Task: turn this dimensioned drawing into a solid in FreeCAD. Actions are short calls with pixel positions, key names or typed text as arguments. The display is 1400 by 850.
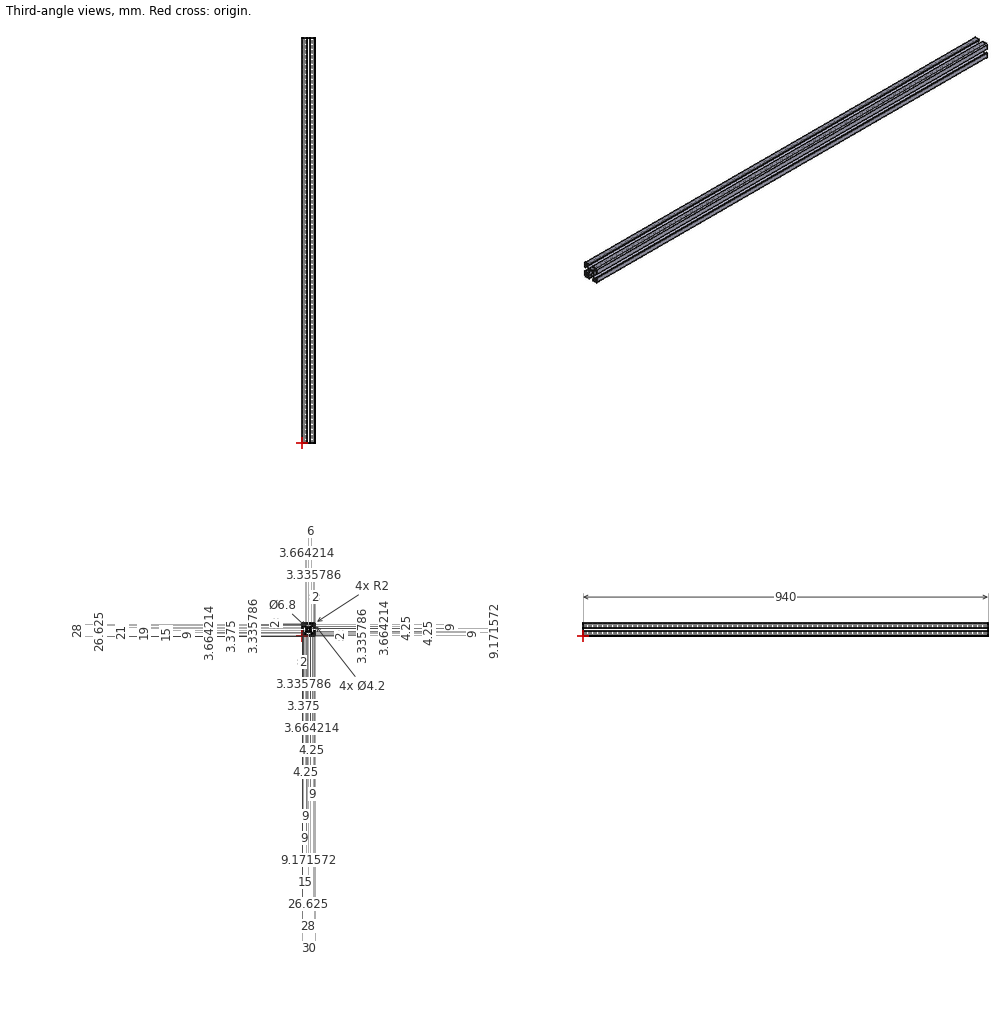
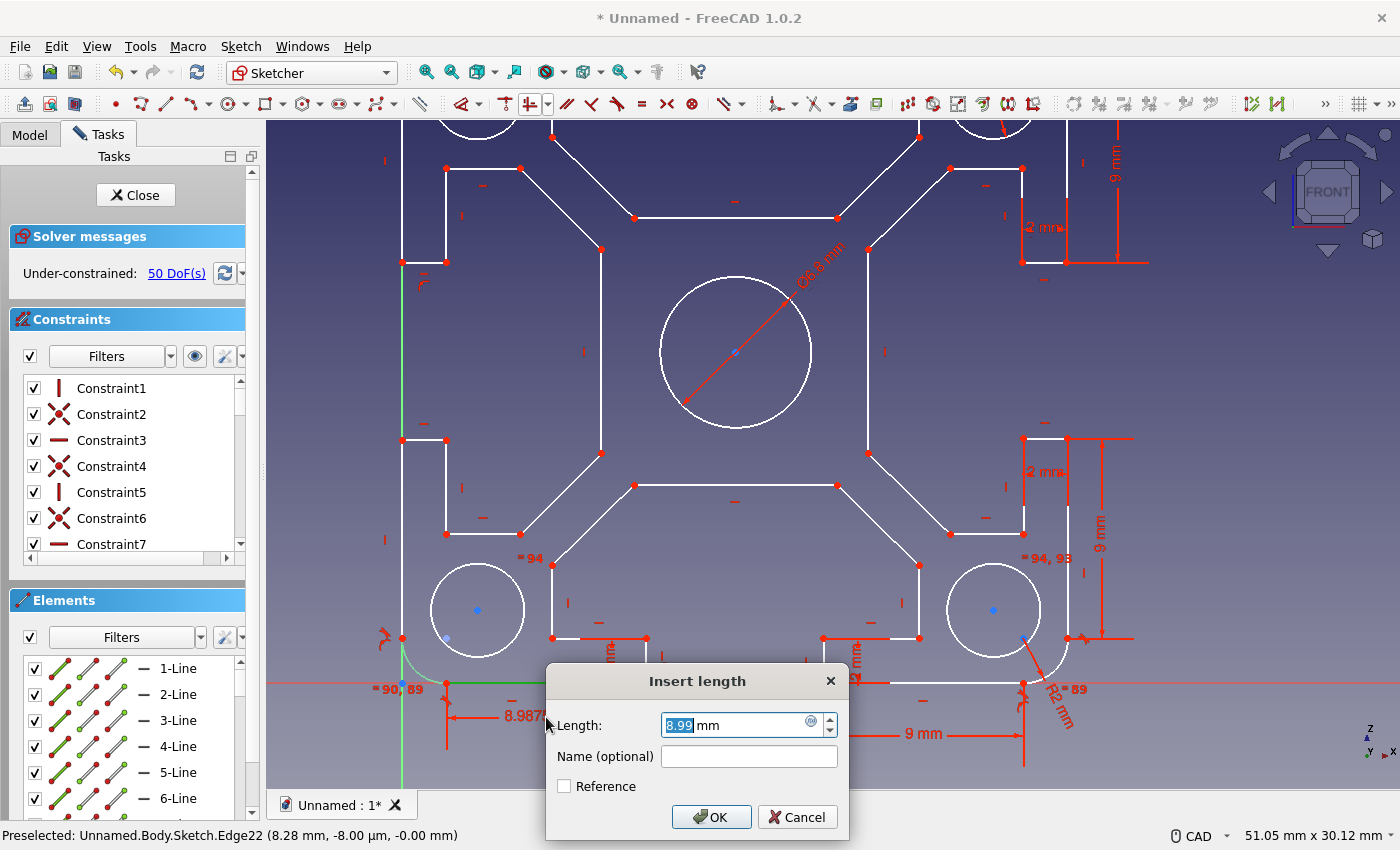
text(9)
key(Return)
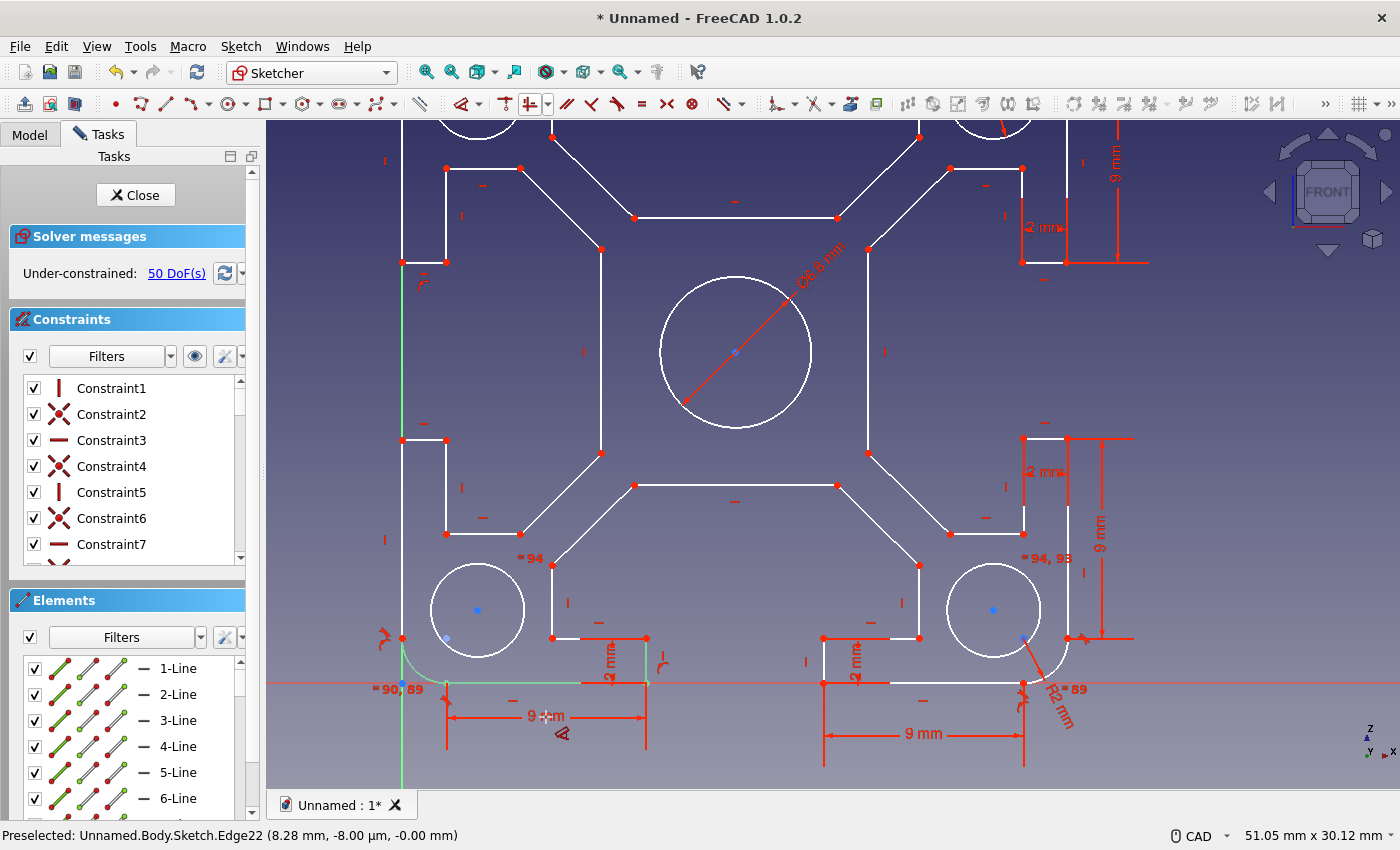
click(402, 579)
click(368, 540)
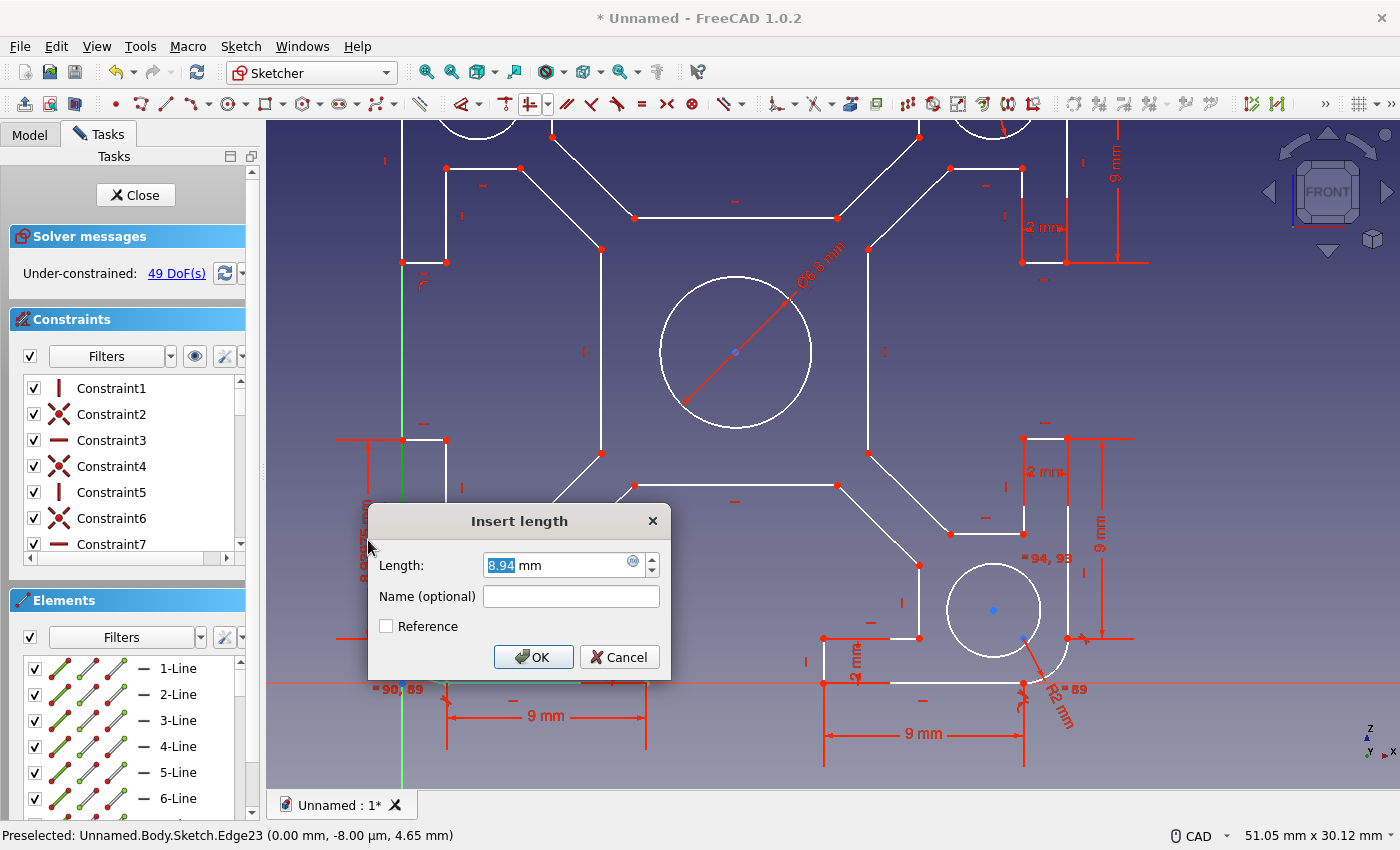
text(9)
key(Return)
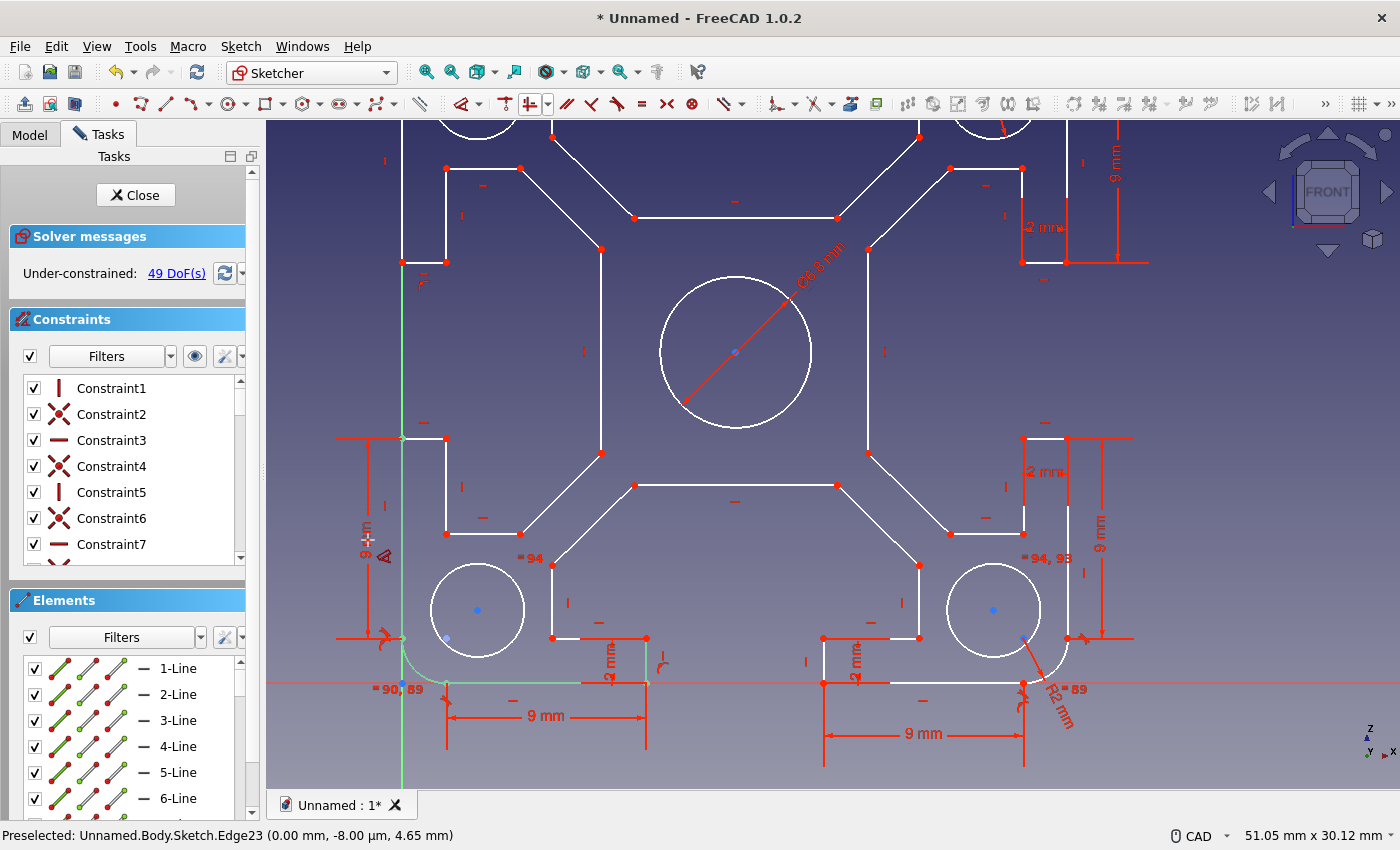
click(415, 439)
click(424, 473)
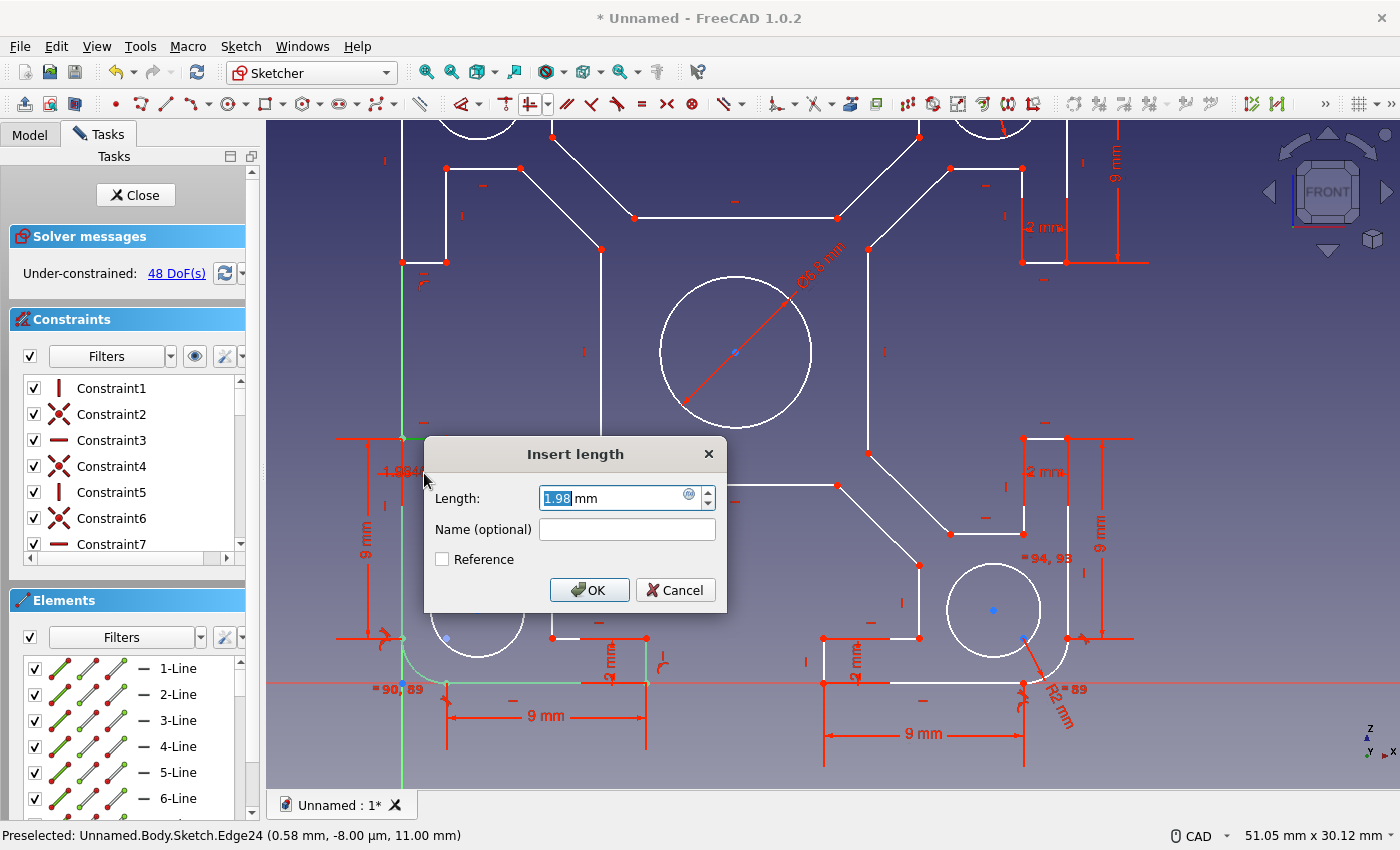
text(2)
key(Return)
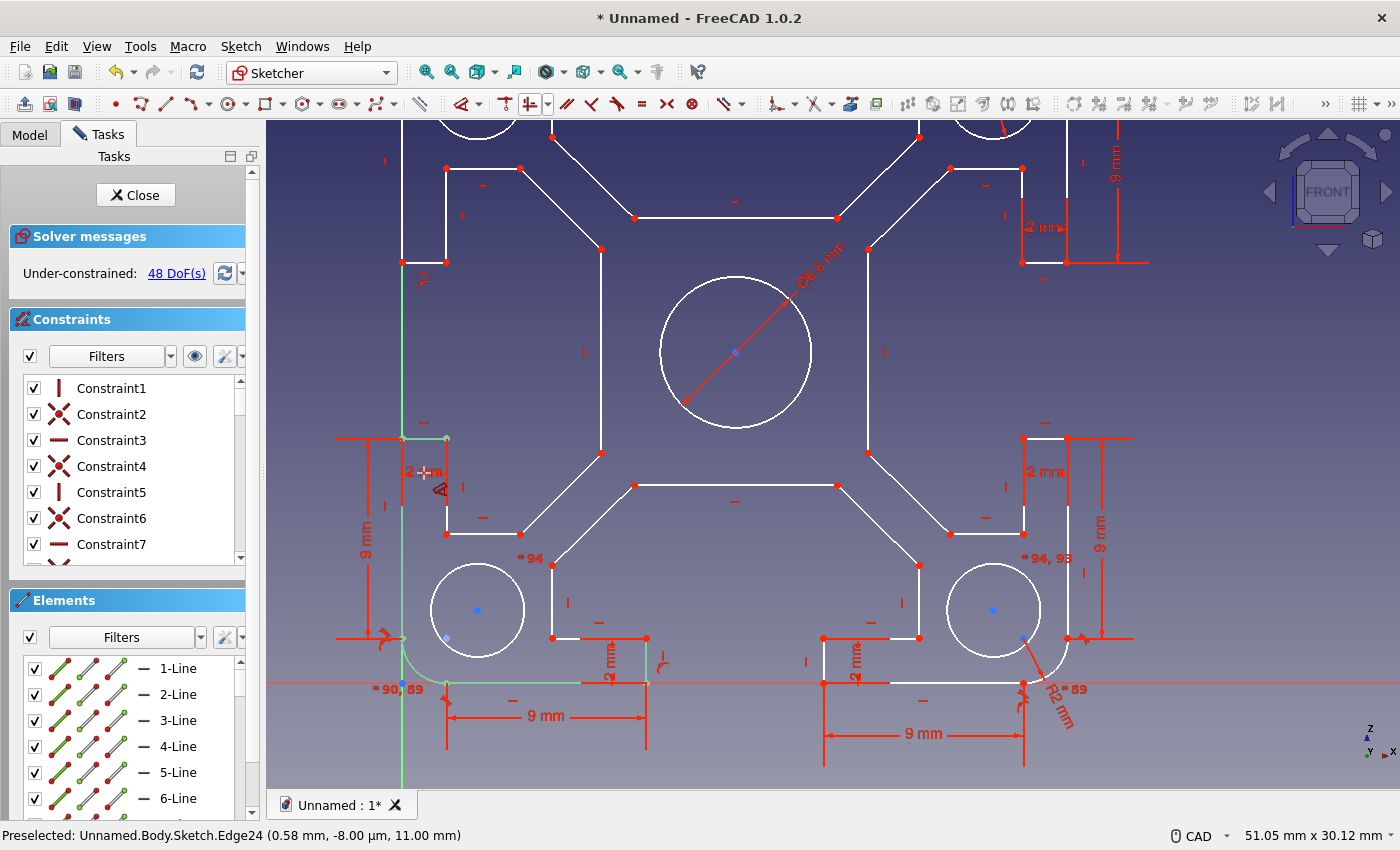
click(433, 263)
click(424, 229)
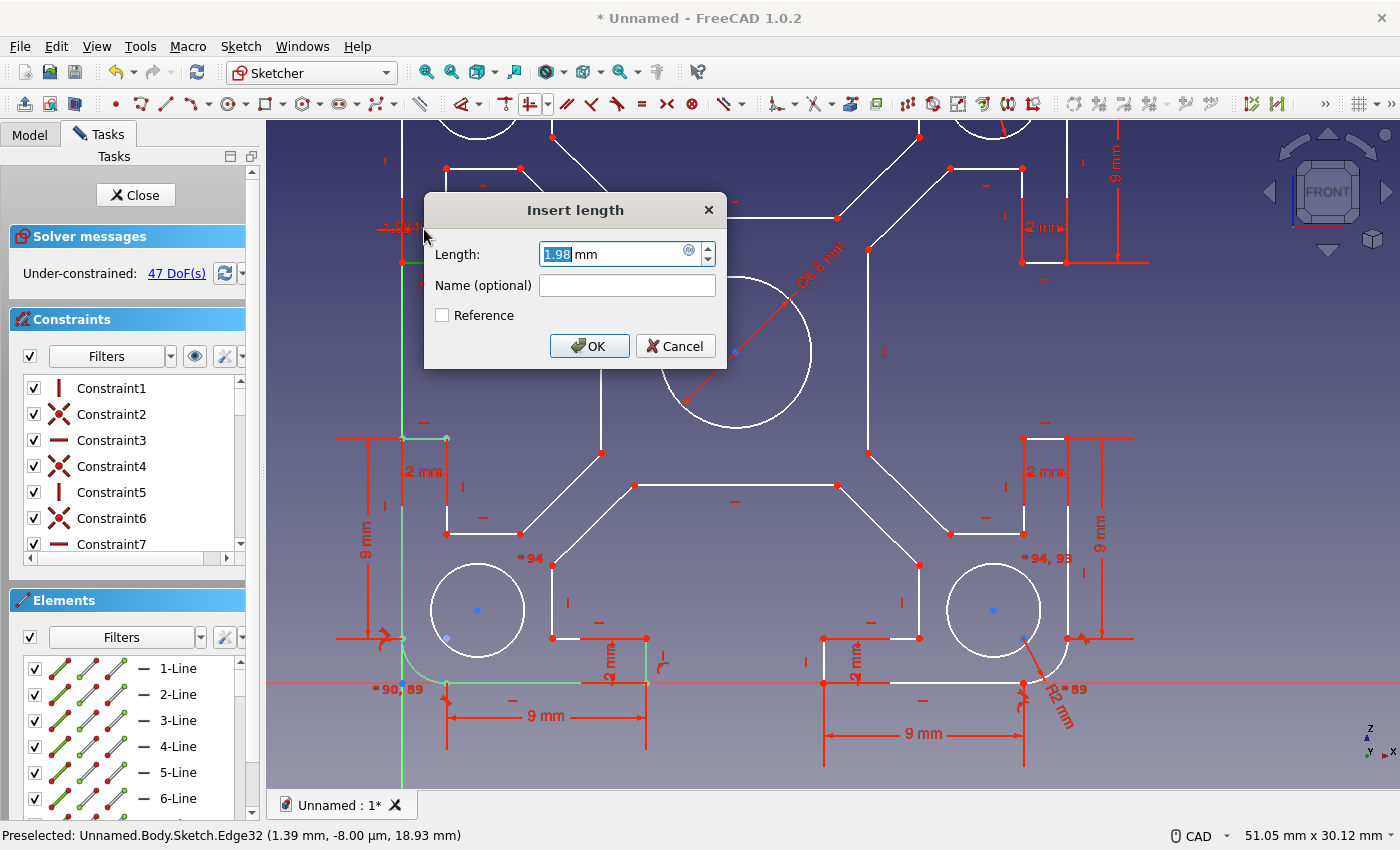
text(2)
key(Return)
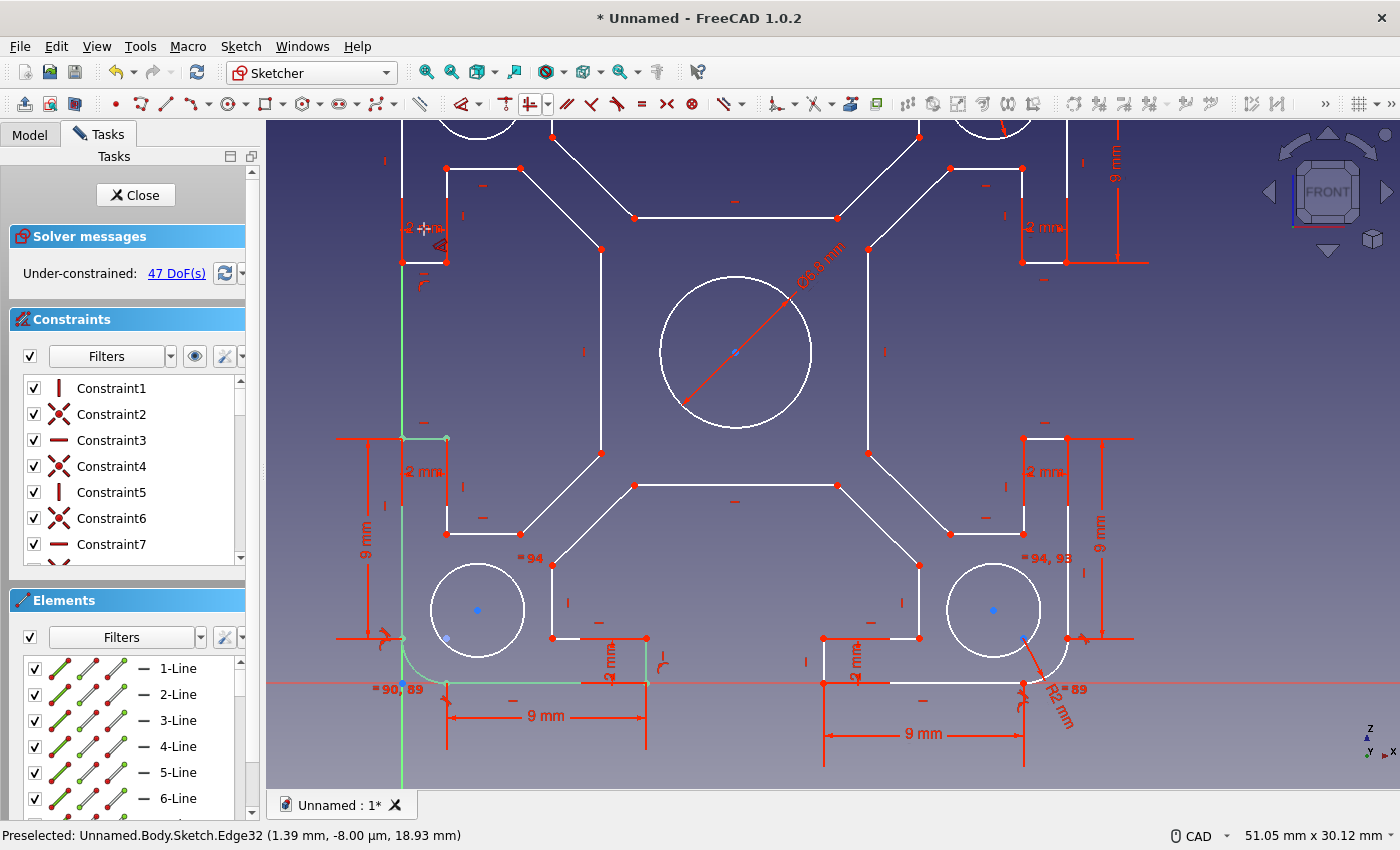
click(402, 201)
click(368, 205)